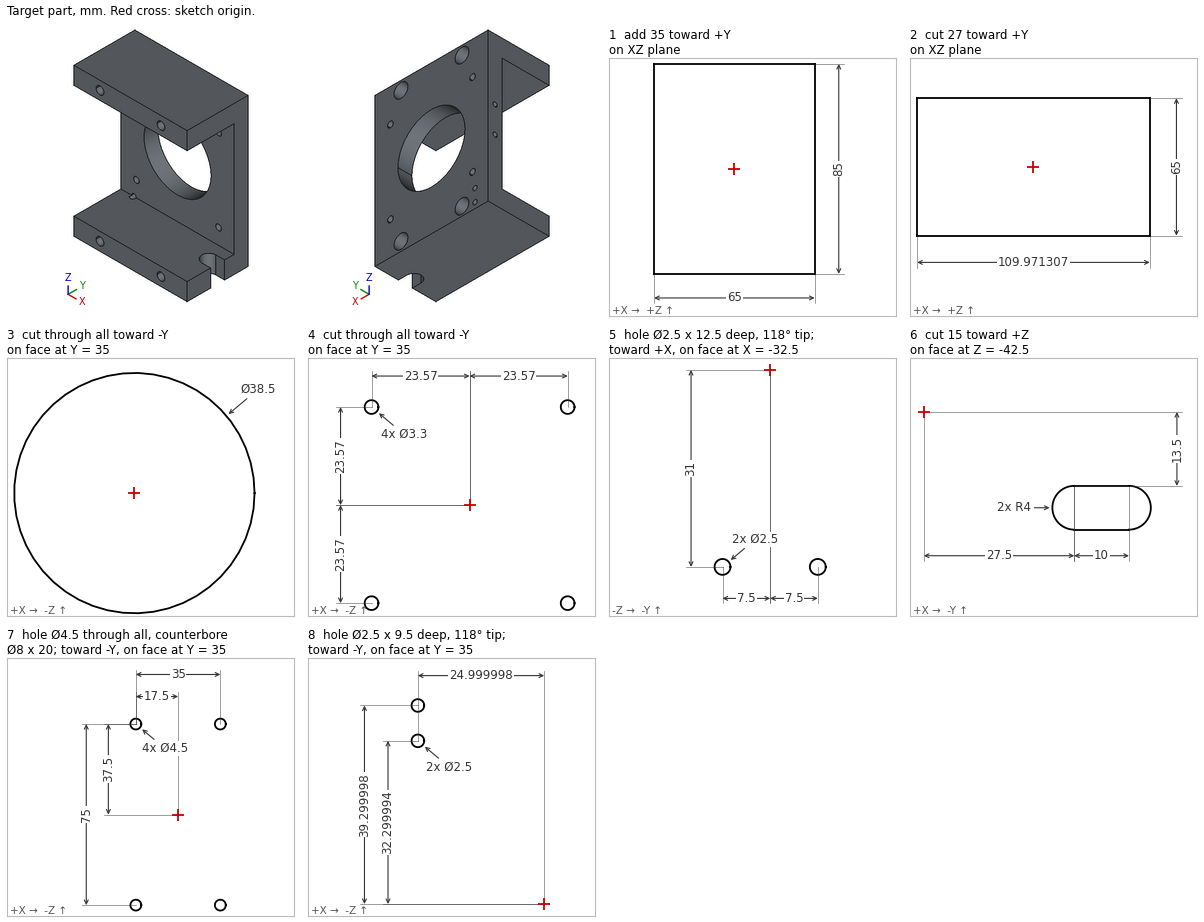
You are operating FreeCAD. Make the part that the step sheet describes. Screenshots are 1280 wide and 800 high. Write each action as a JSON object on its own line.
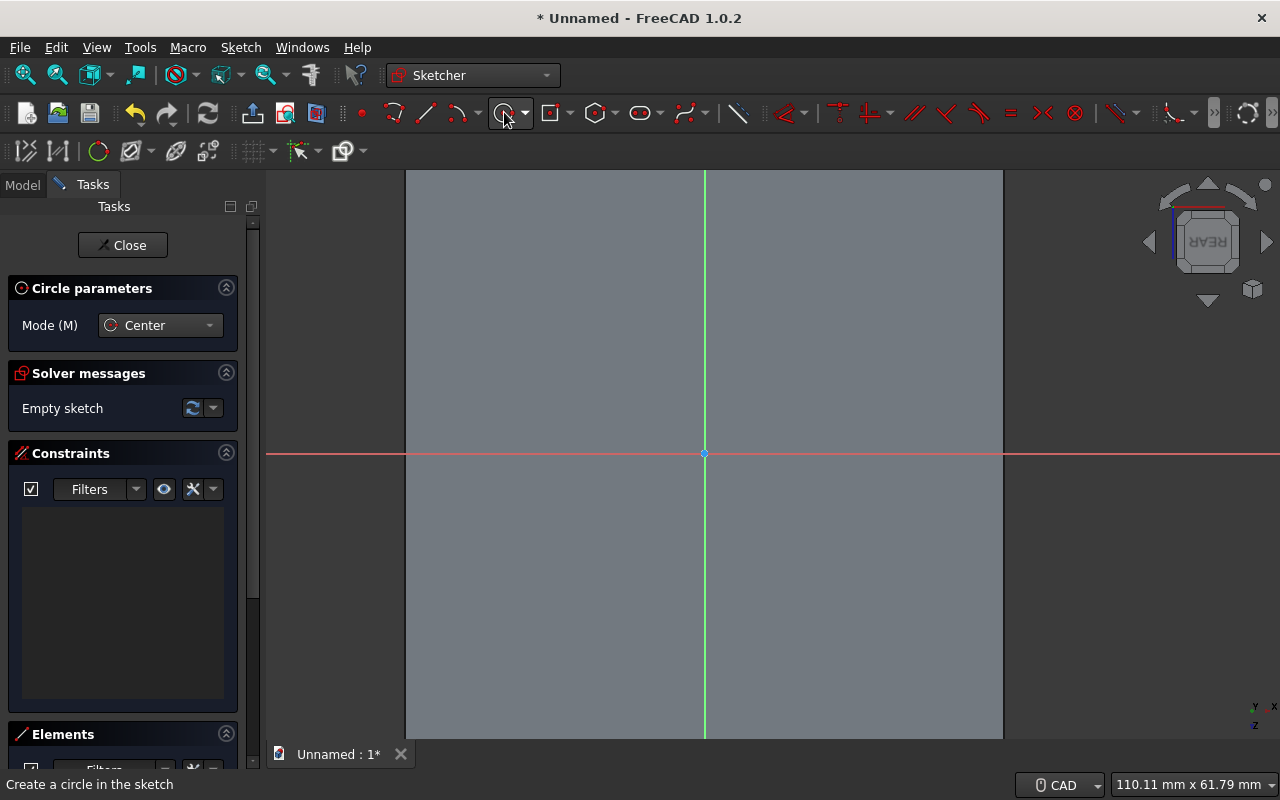
{"action": "left_click", "coordinate": [705, 454]}
{"action": "mouse_move", "coordinate": [830, 328]}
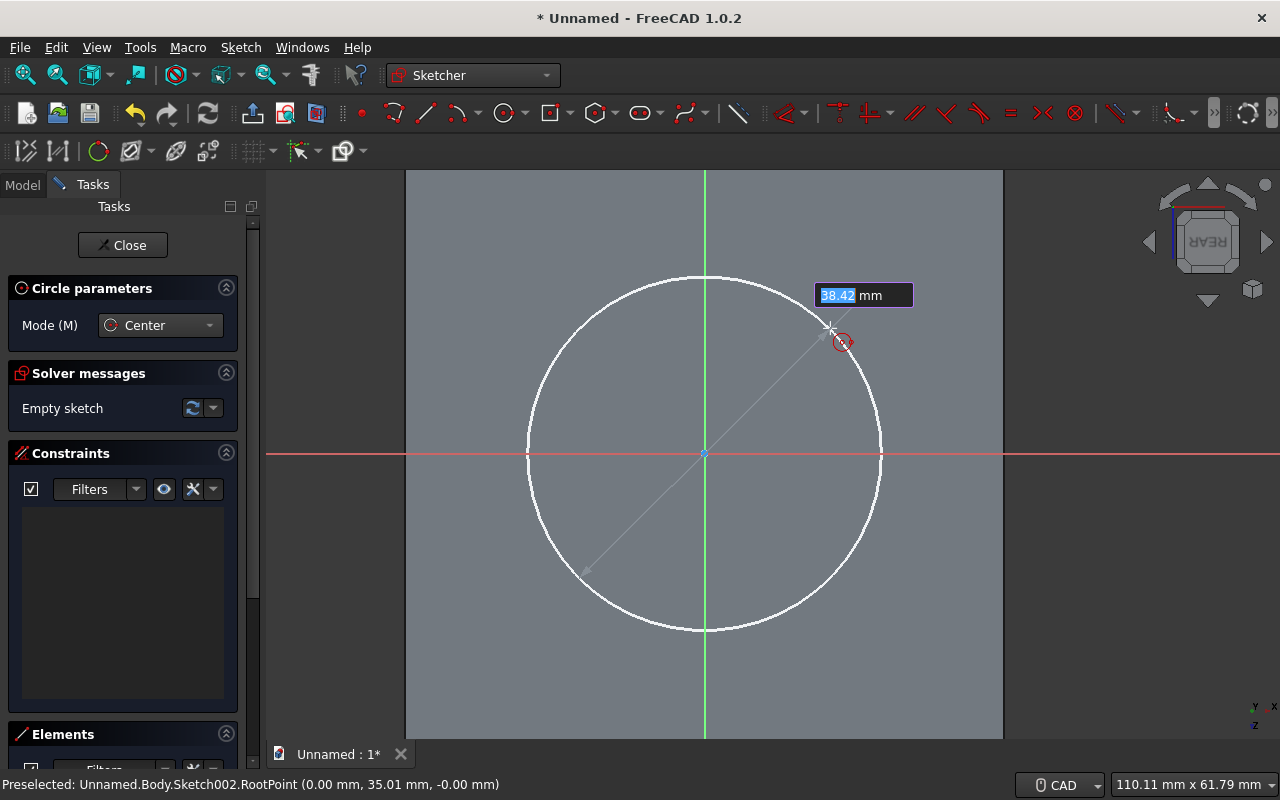
{"action": "type", "text": "38.5"}
{"action": "key", "text": "Return"}
{"action": "key", "text": "Escape"}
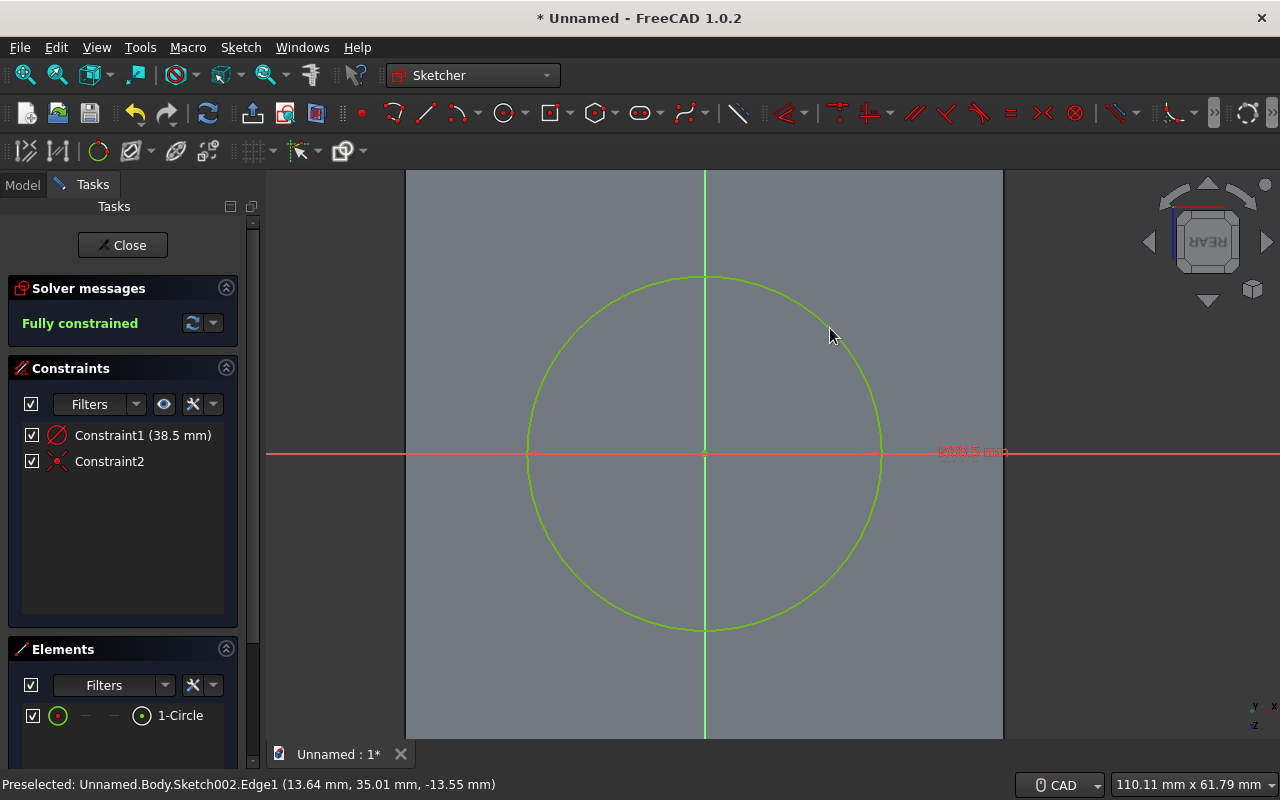
{"action": "left_click", "coordinate": [123, 245]}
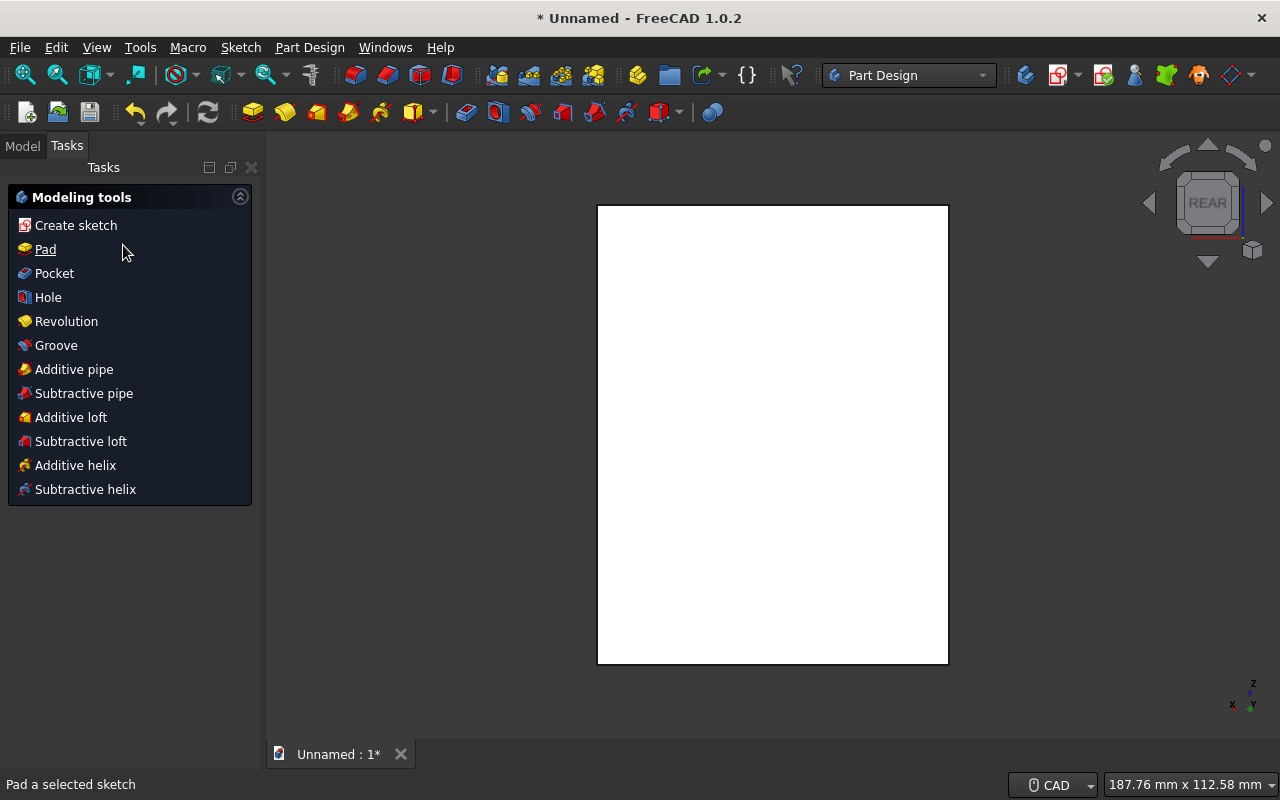
{"action": "left_click", "coordinate": [468, 112]}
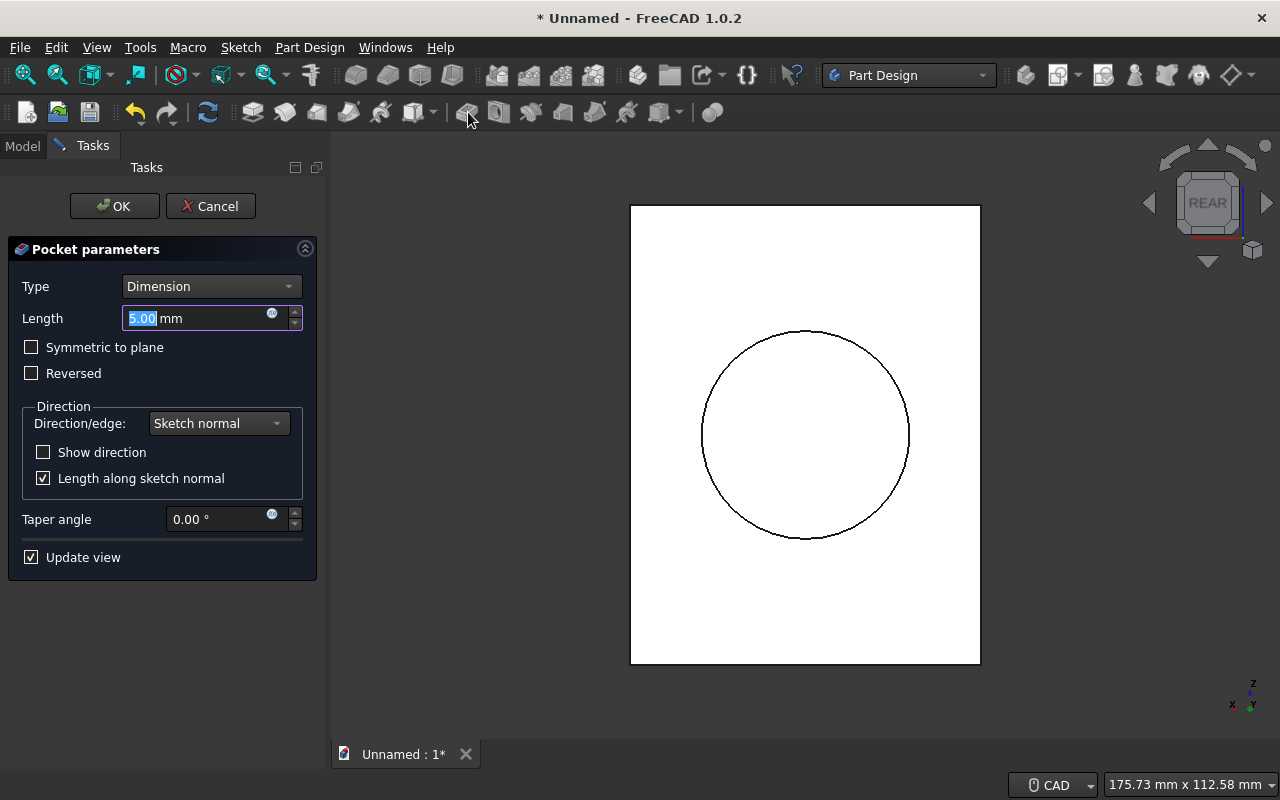
{"action": "left_click", "coordinate": [212, 286]}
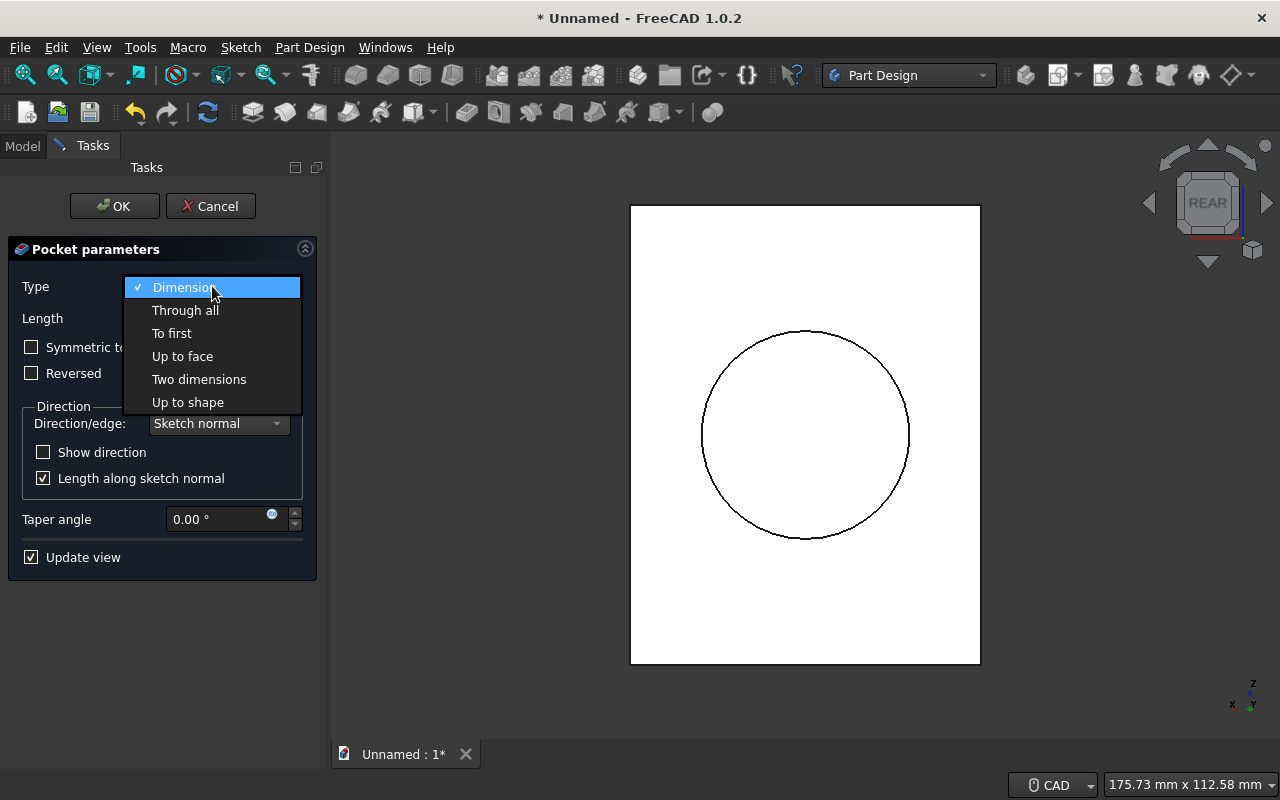
{"action": "left_click", "coordinate": [212, 310]}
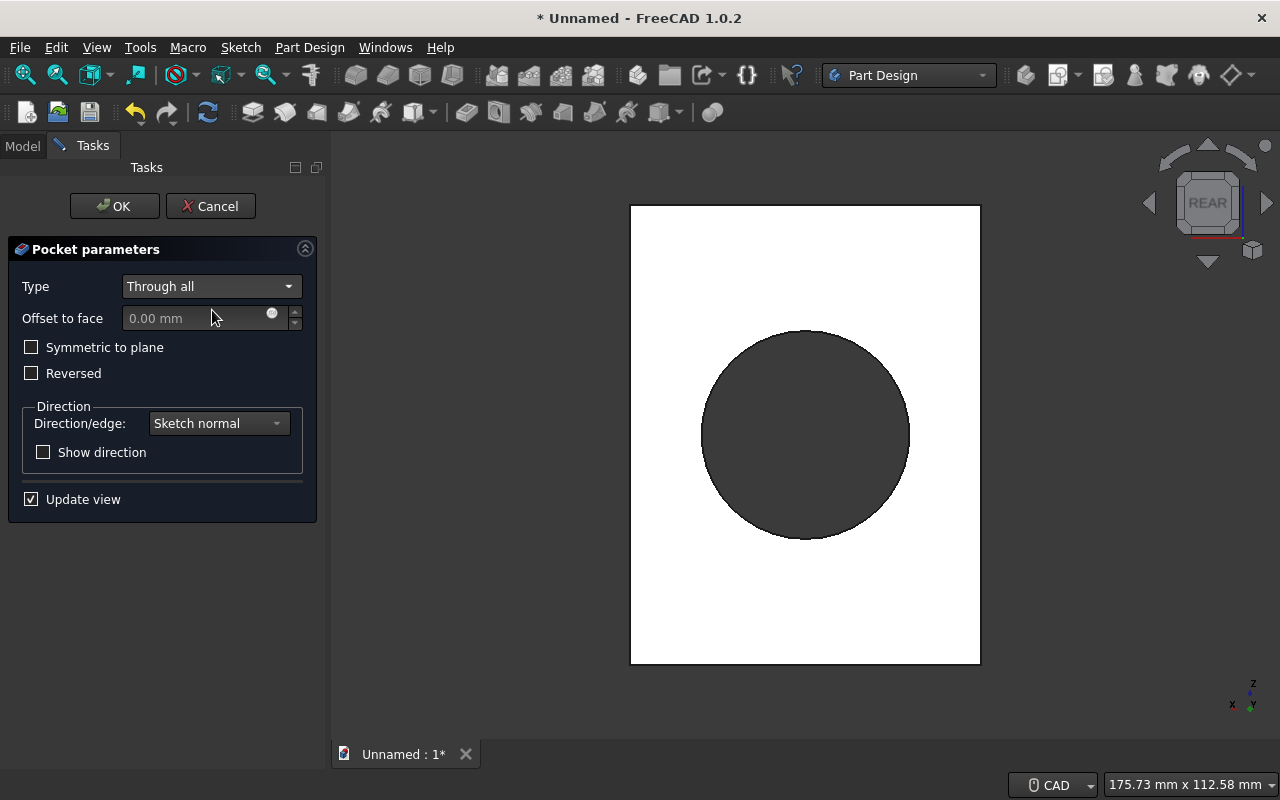
{"action": "left_click", "coordinate": [115, 206]}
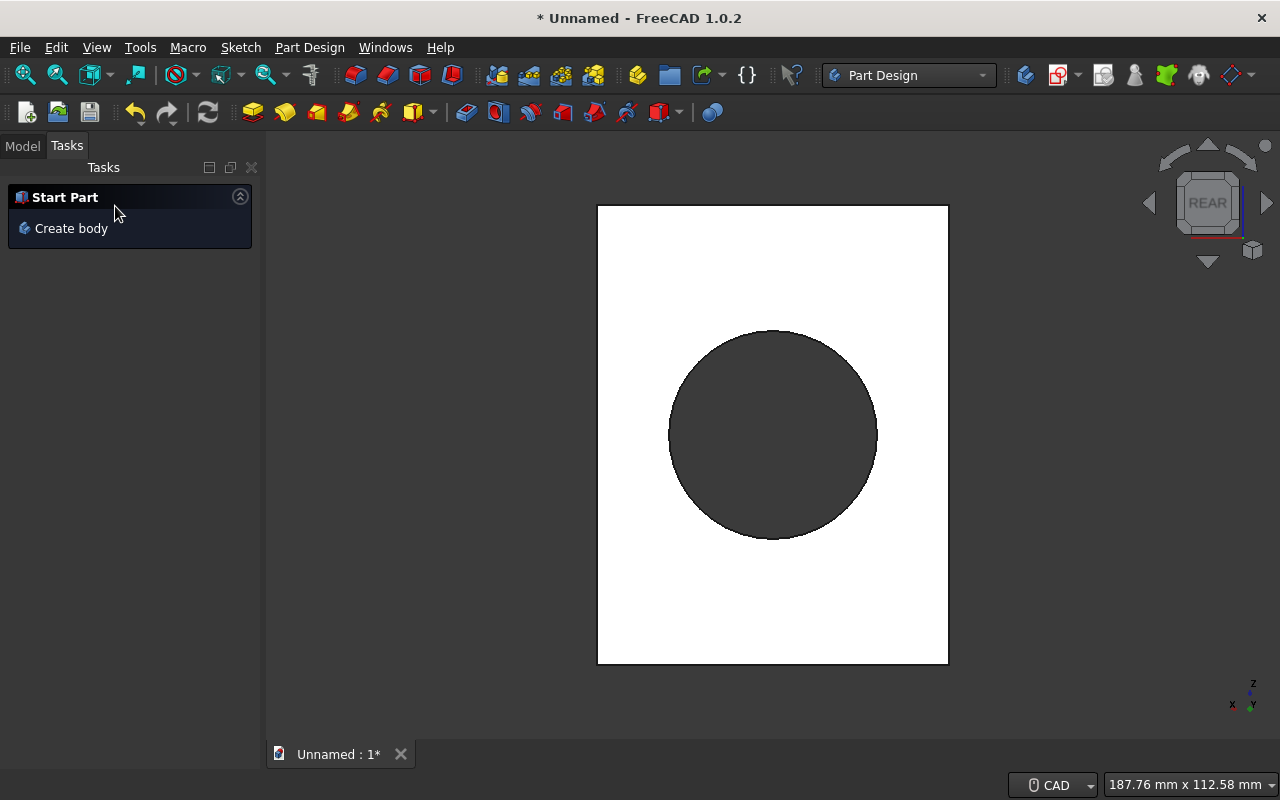
{"action": "left_click", "coordinate": [673, 565]}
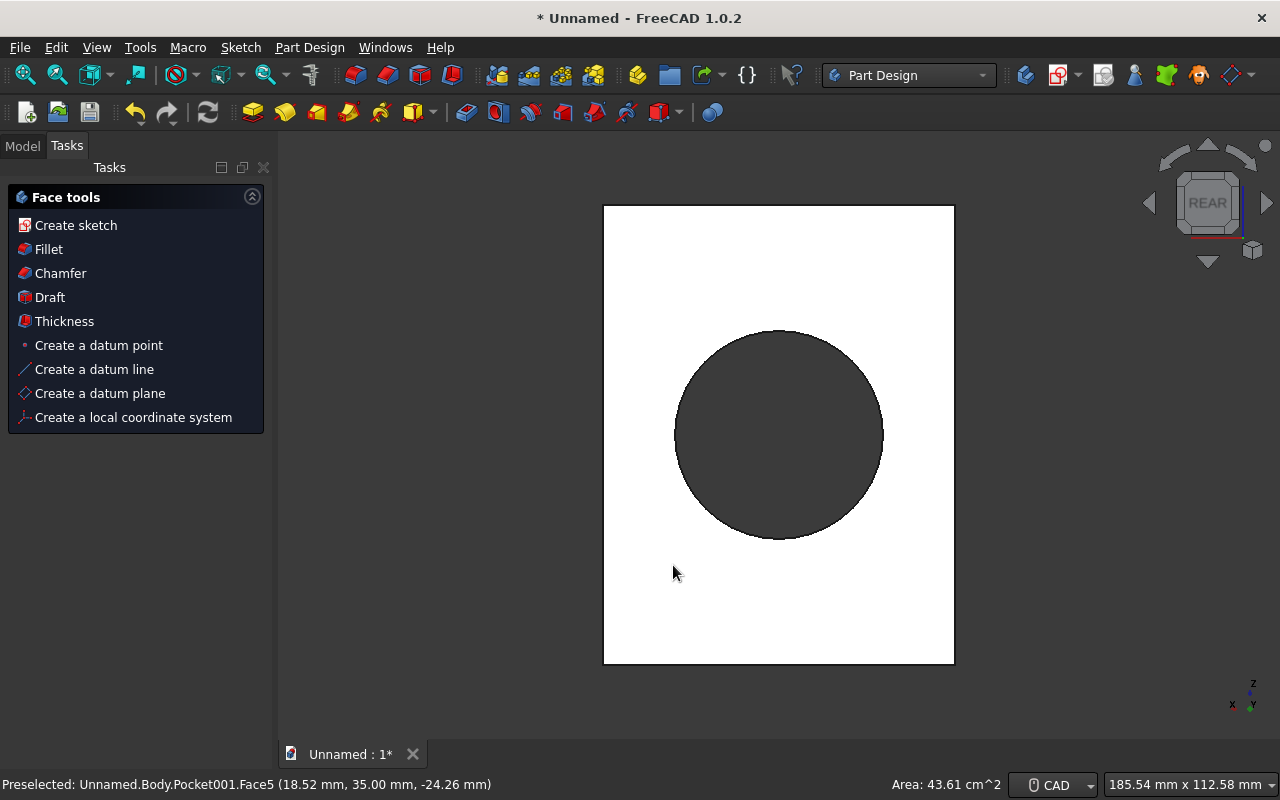
{"action": "left_click", "coordinate": [1058, 76]}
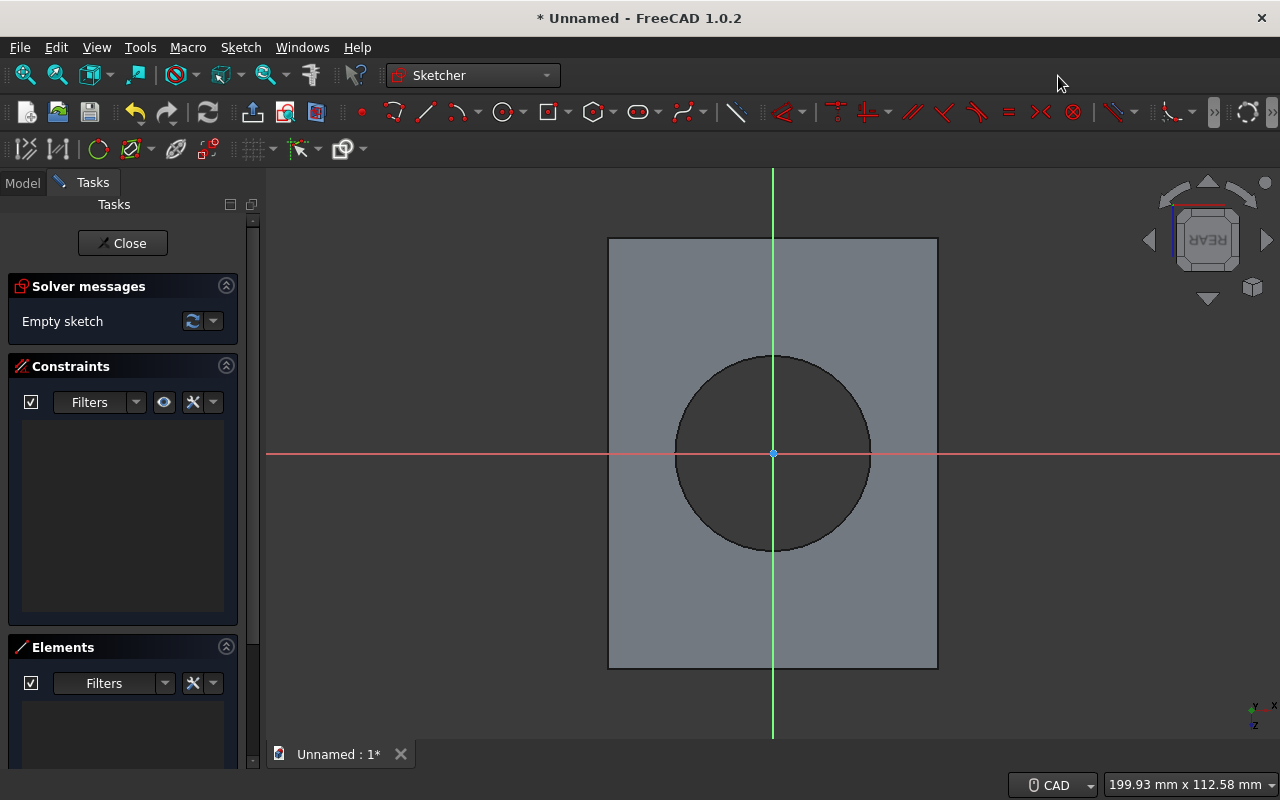
{"action": "scroll", "coordinate": [912, 453], "scroll_direction": "up", "scroll_amount": 2}